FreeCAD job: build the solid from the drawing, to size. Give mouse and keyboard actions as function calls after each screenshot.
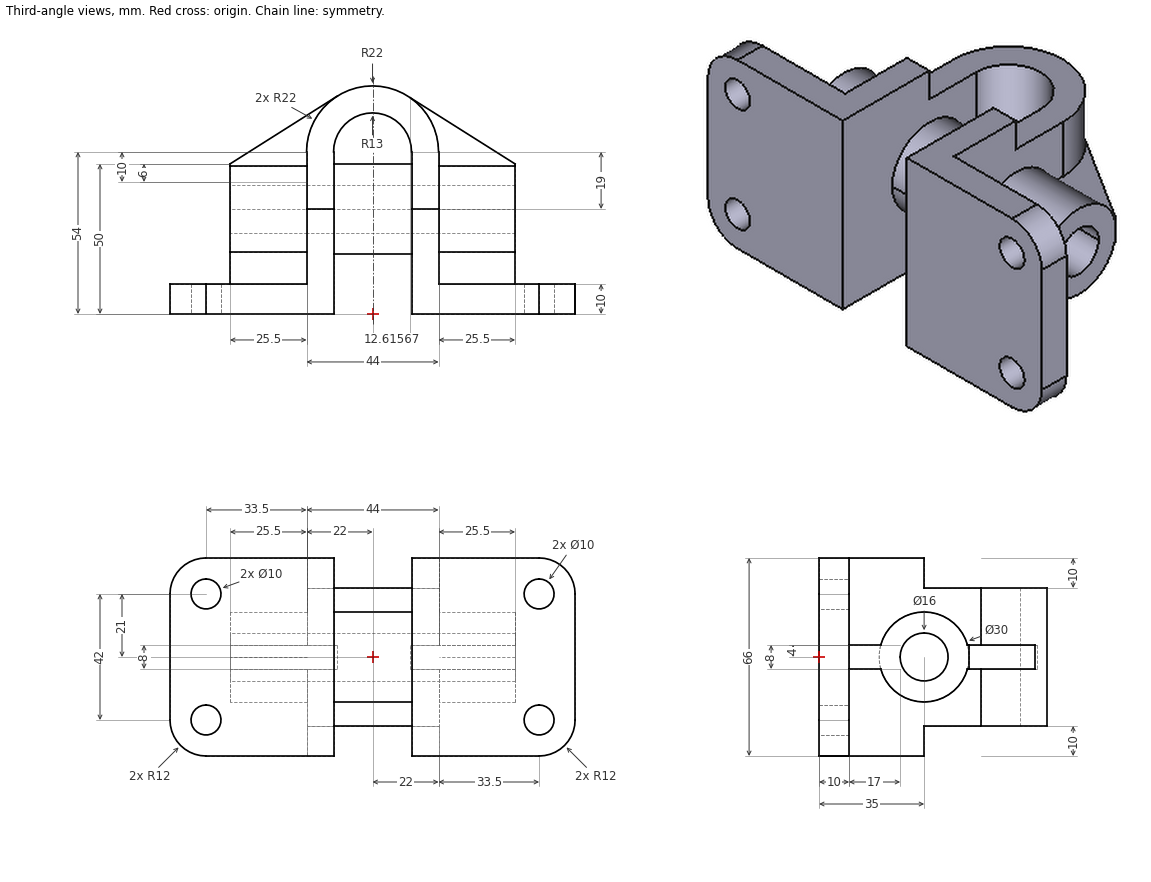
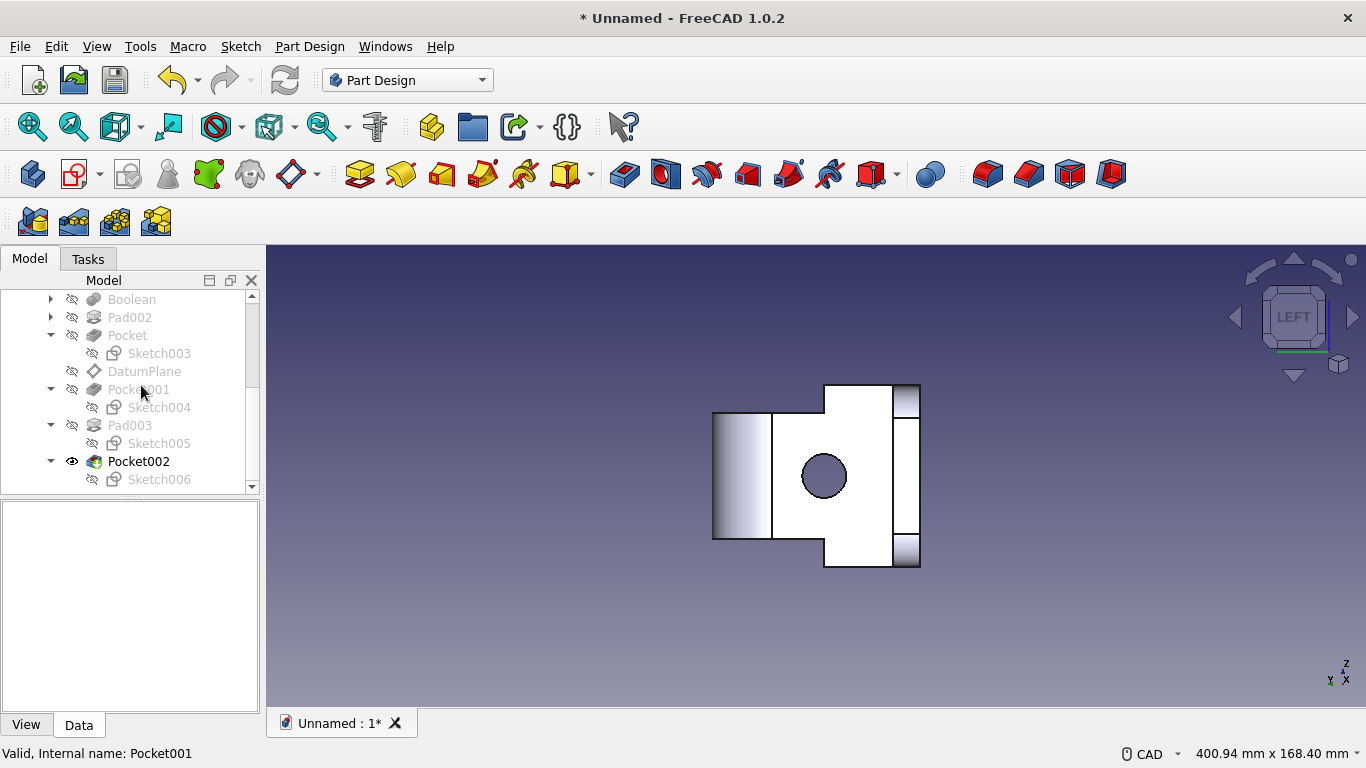
scroll(141, 385, up, 15)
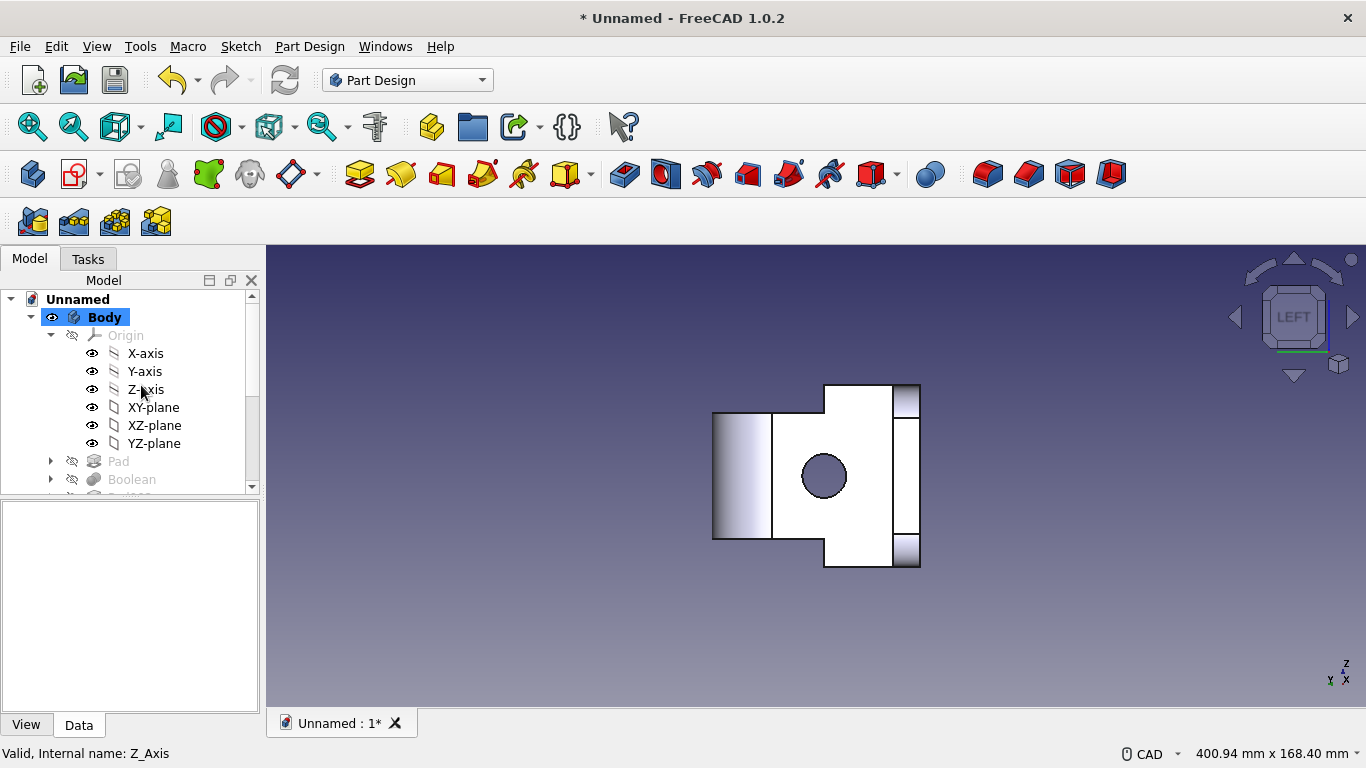
click(137, 443)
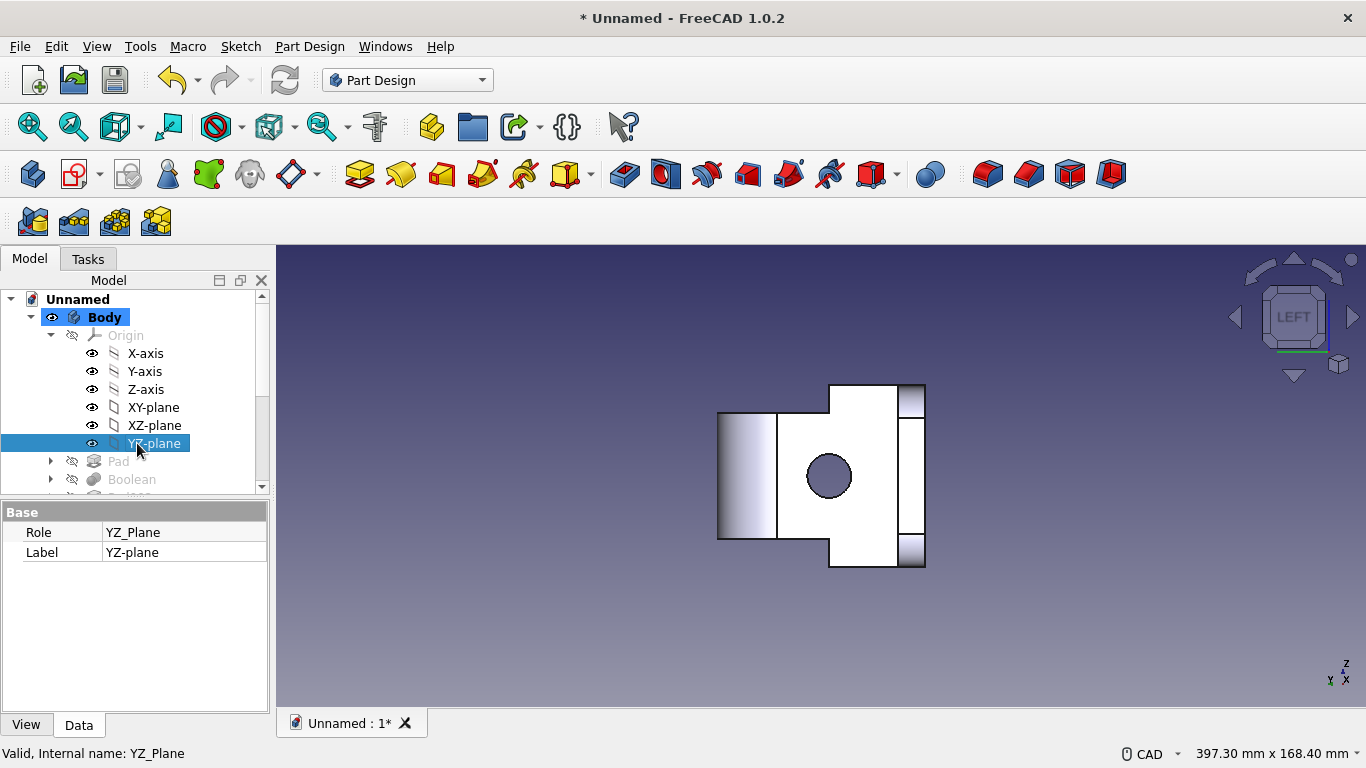
click(290, 174)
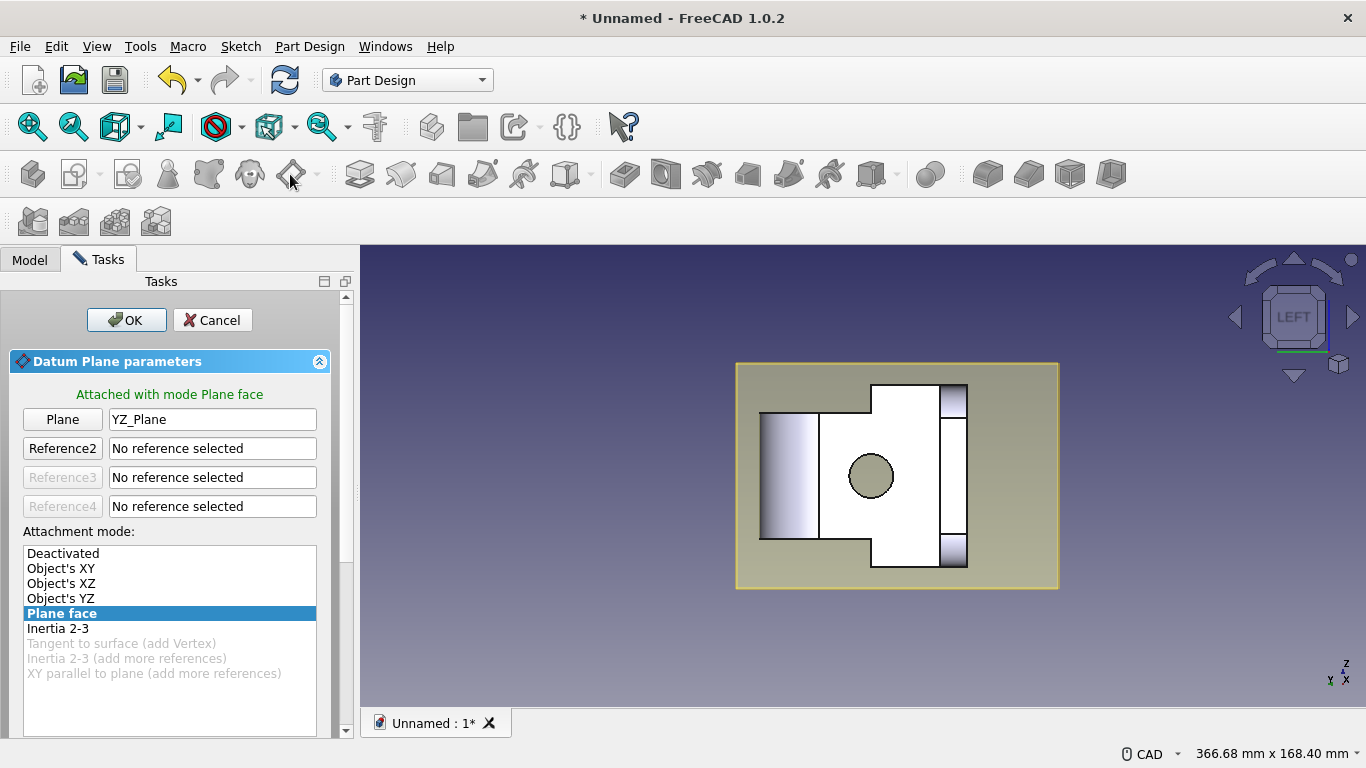
scroll(346, 514, down, 4)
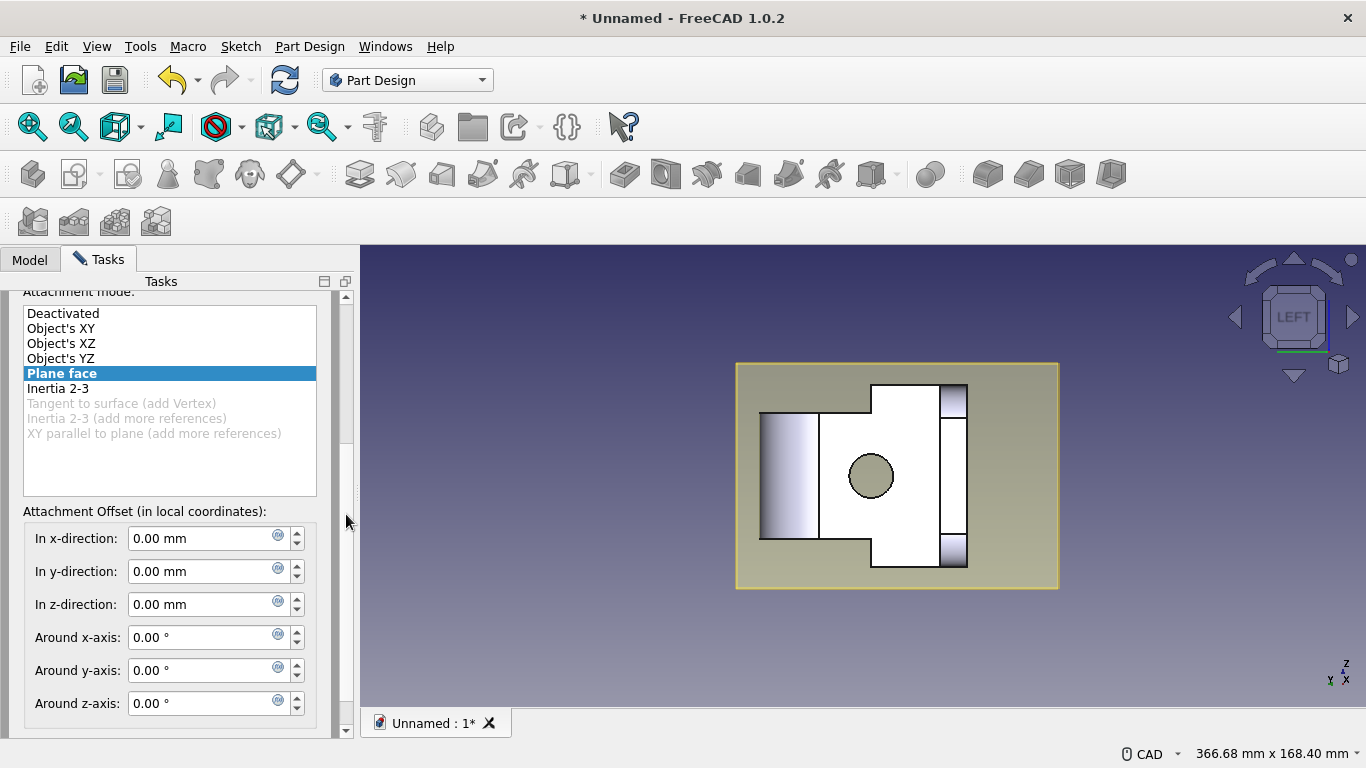
triple_click(210, 604)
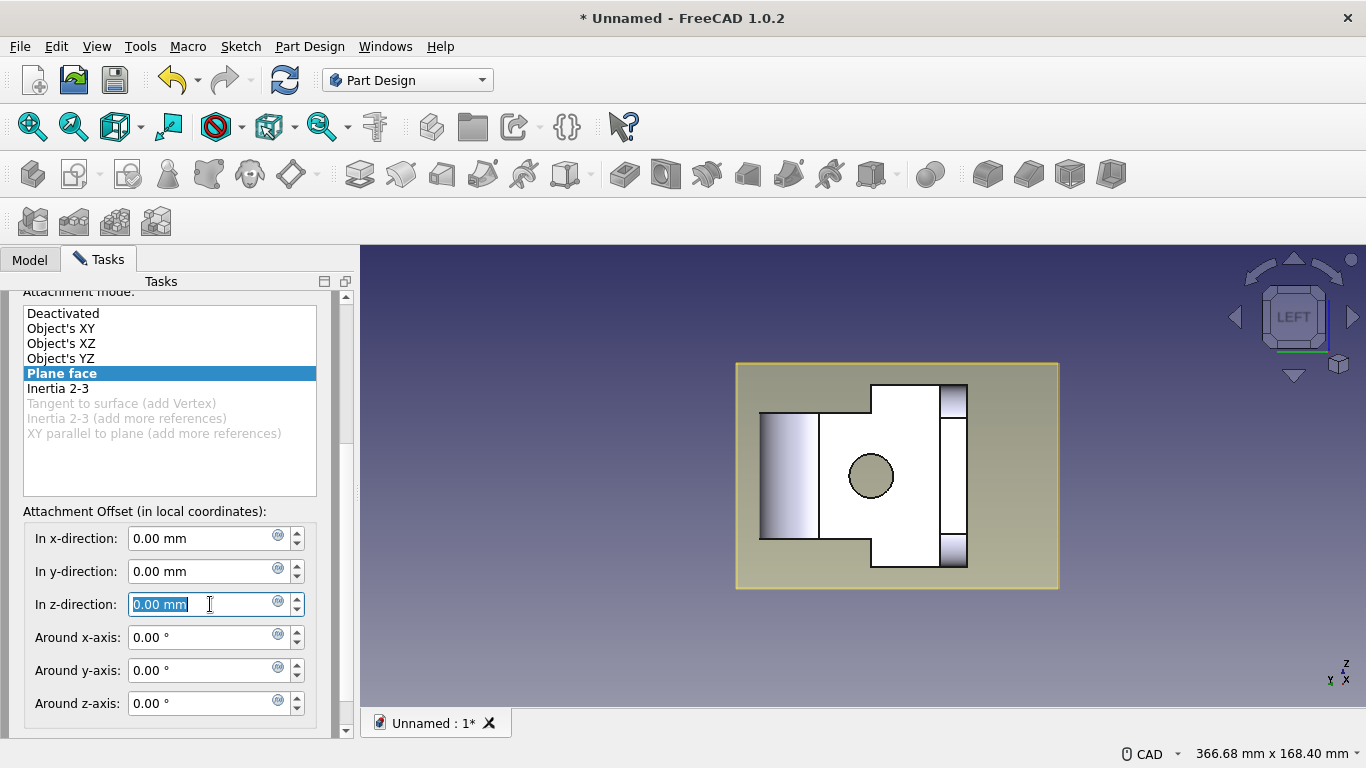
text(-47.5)
key(Tab)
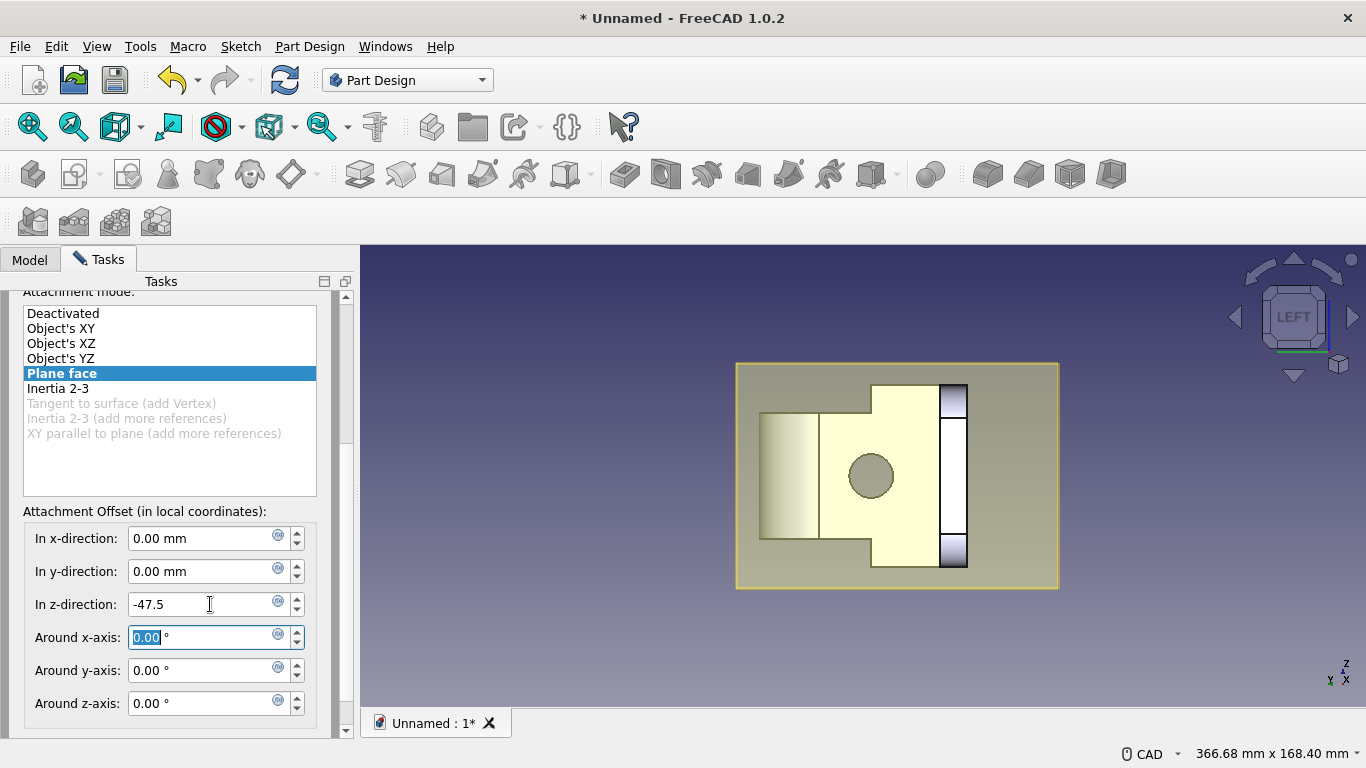
scroll(346, 514, up, 5)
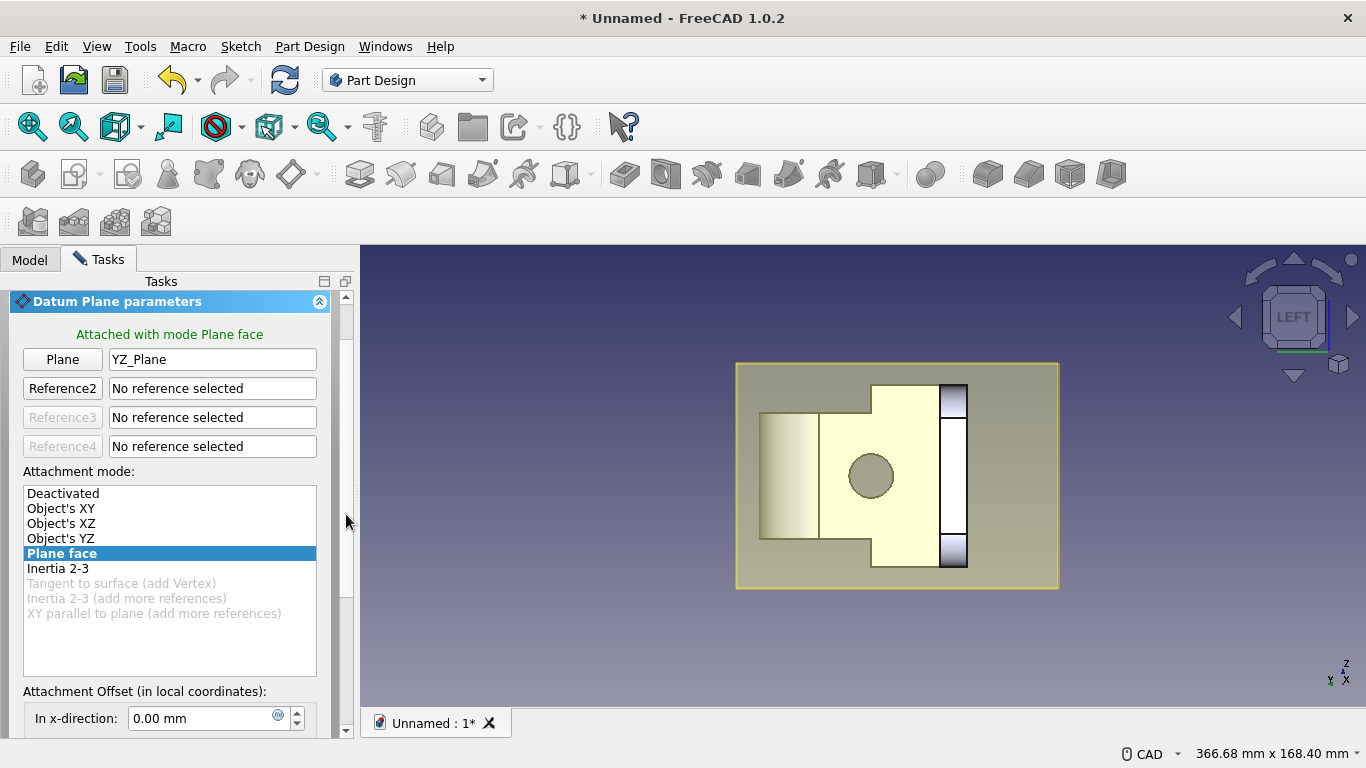
click(127, 320)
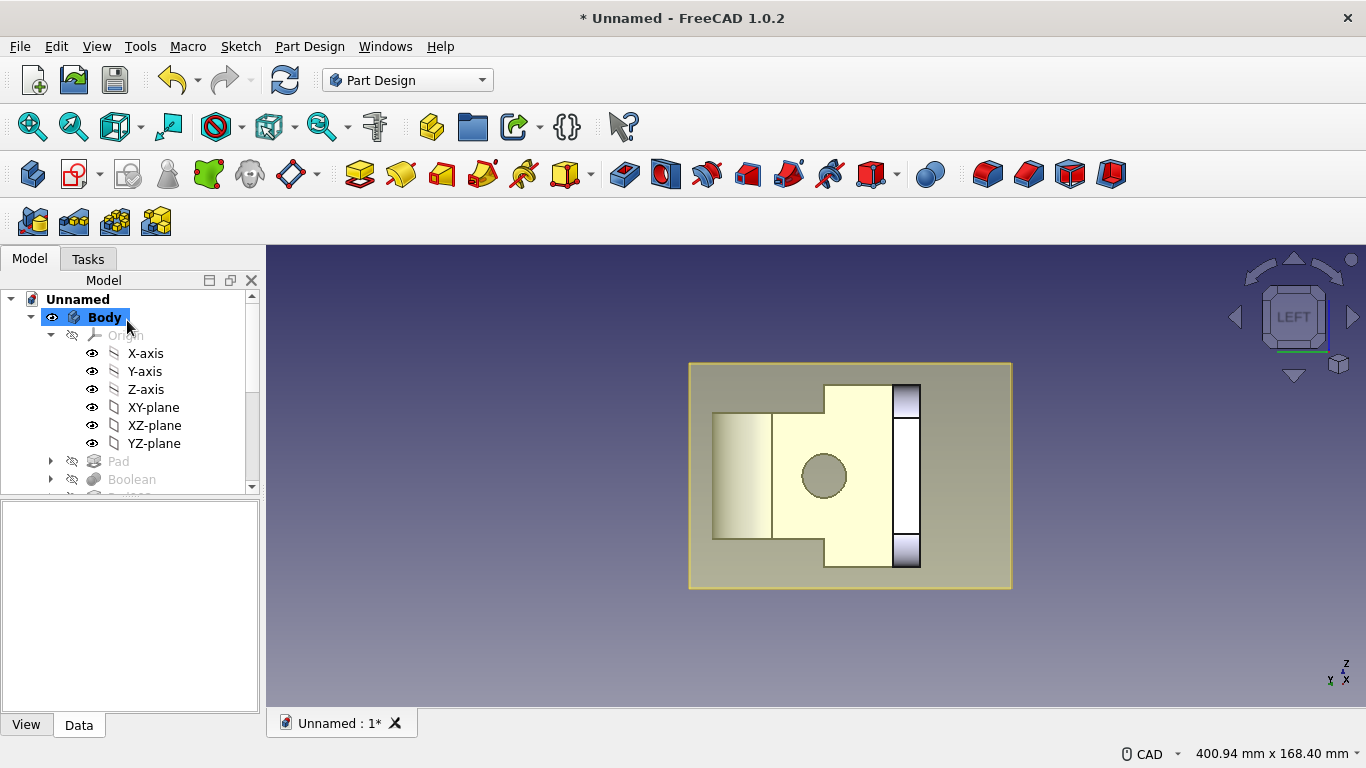
scroll(101, 385, down, 3)